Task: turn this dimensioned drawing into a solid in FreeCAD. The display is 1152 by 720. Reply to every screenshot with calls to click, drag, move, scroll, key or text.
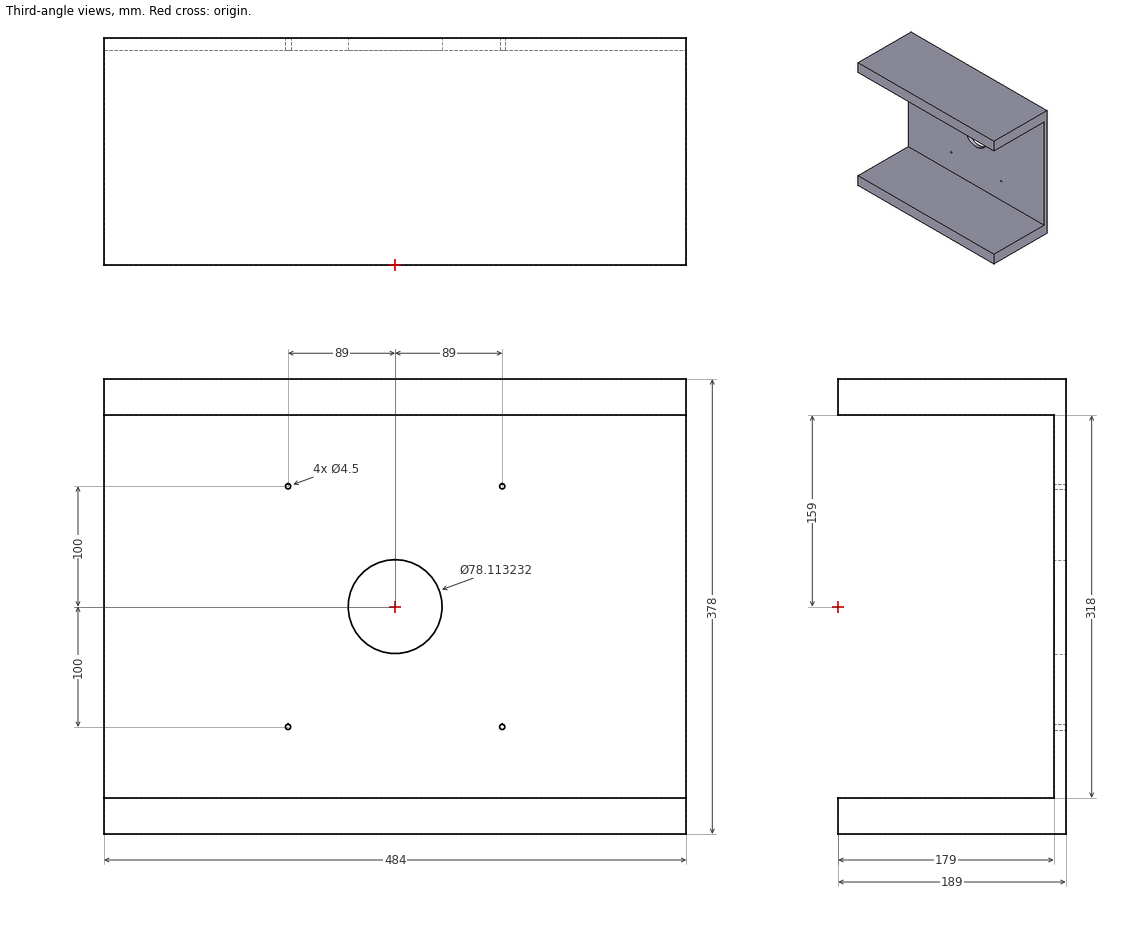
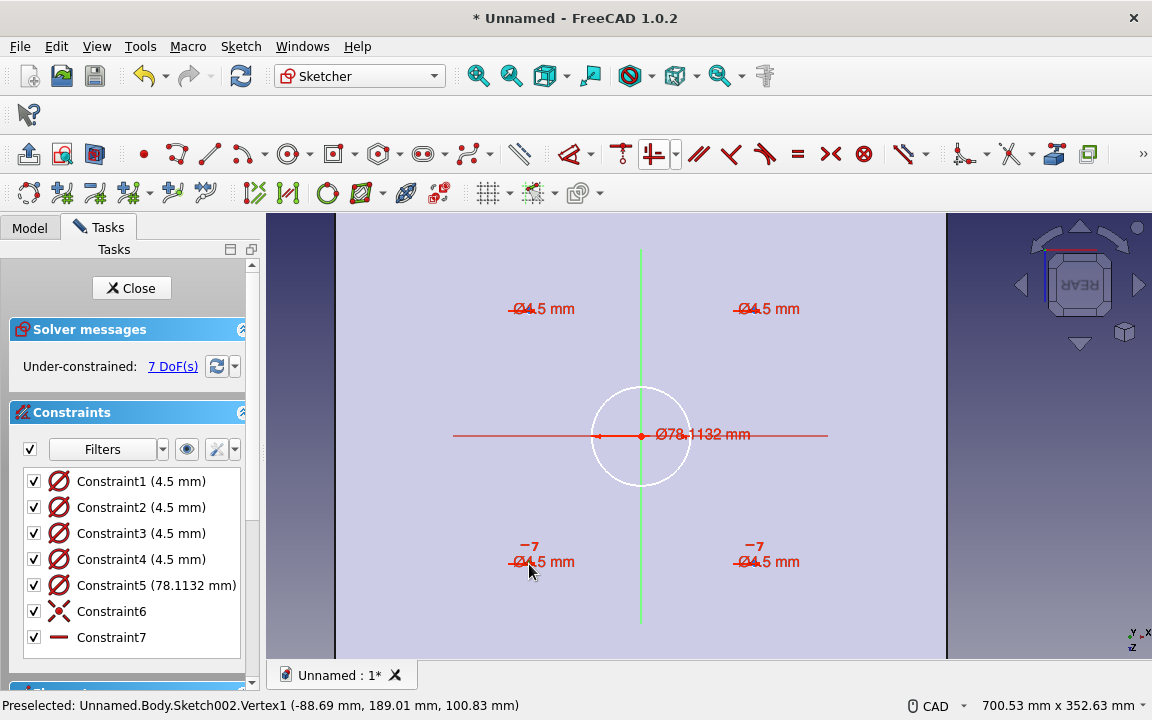
click(529, 311)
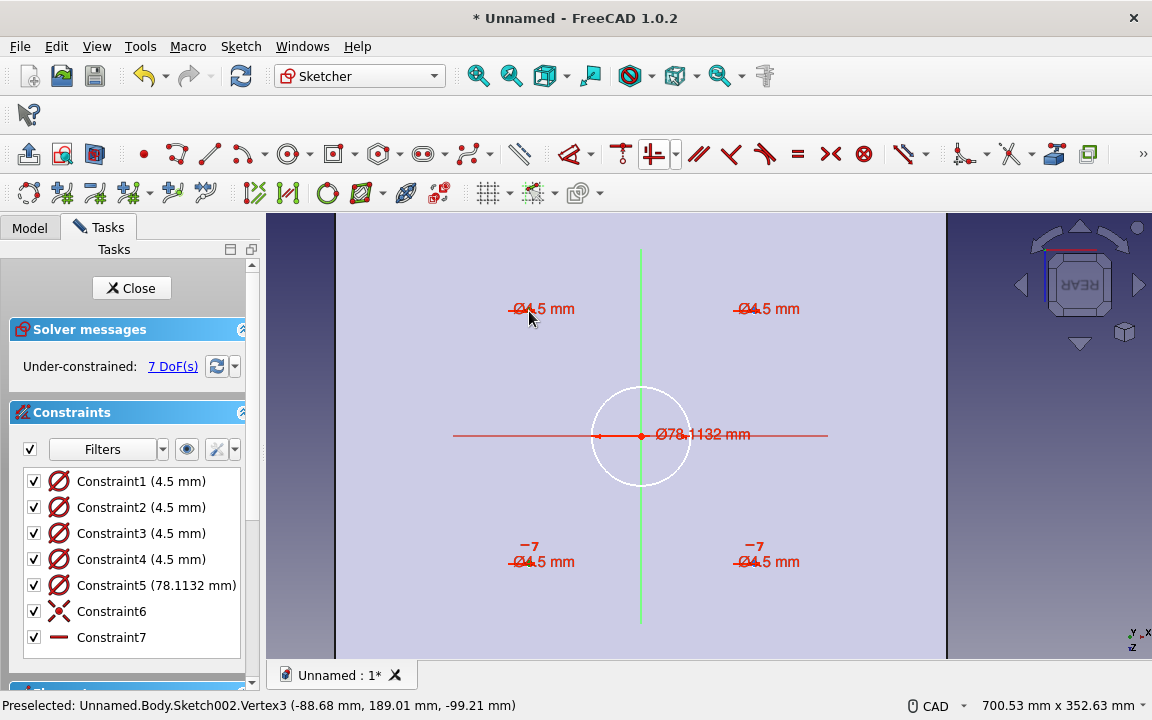
key(v)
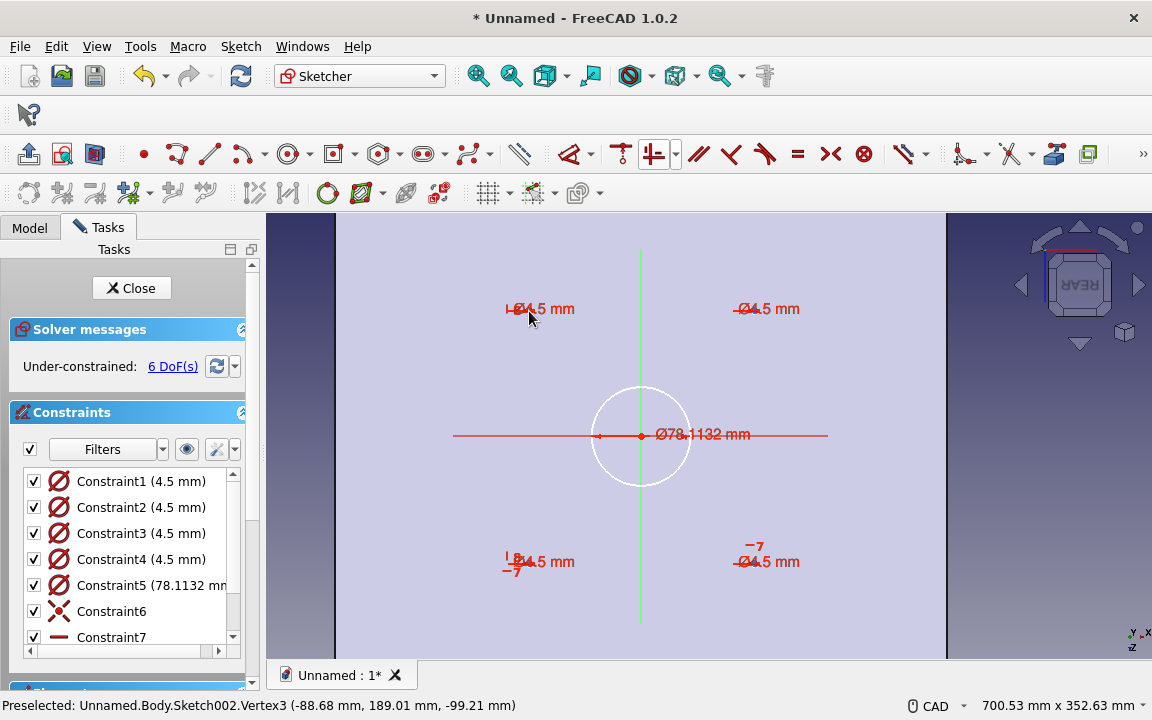
click(754, 564)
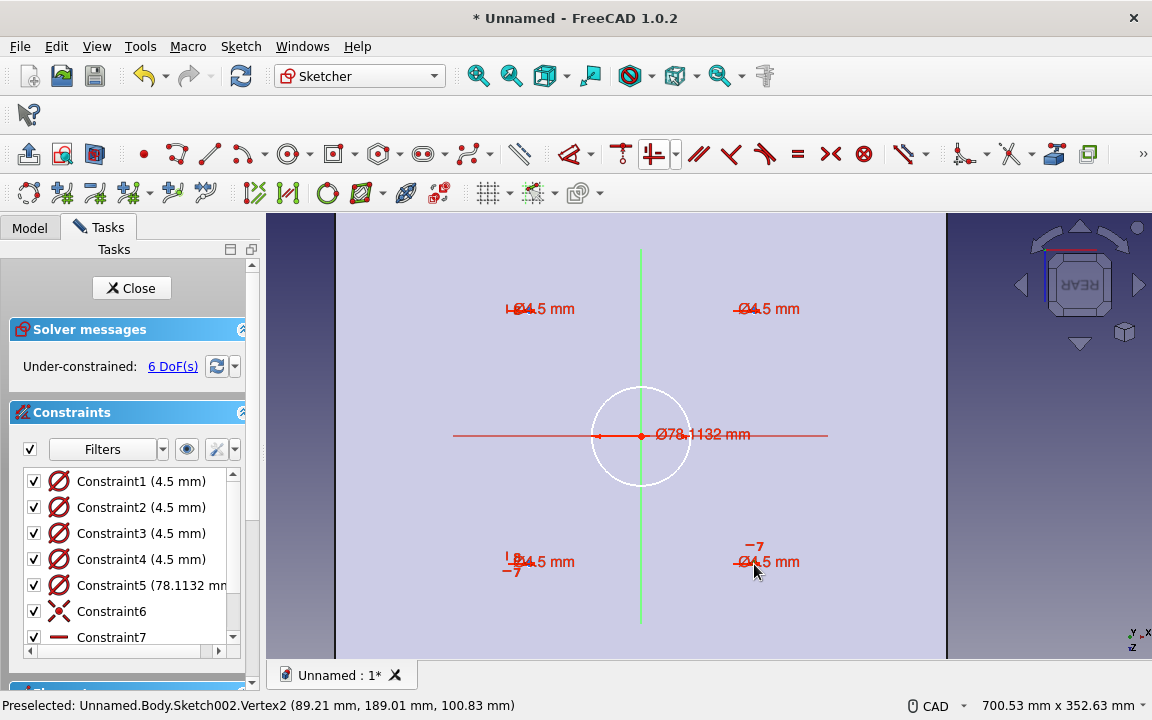
click(754, 311)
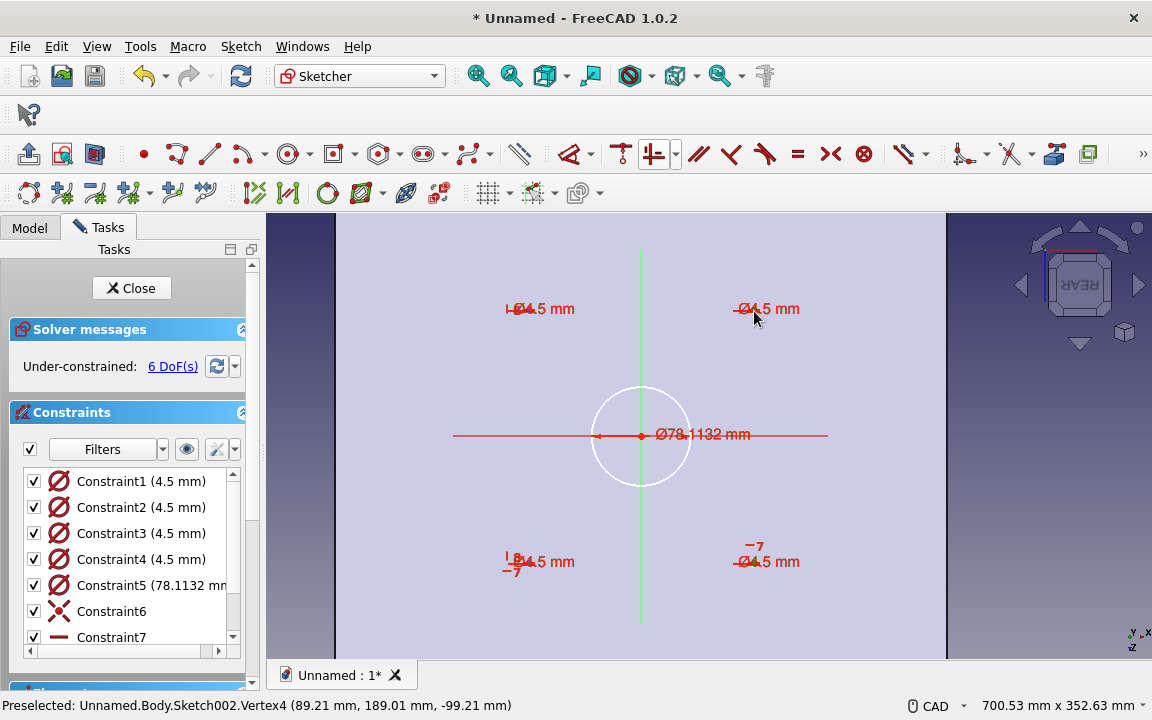
key(v)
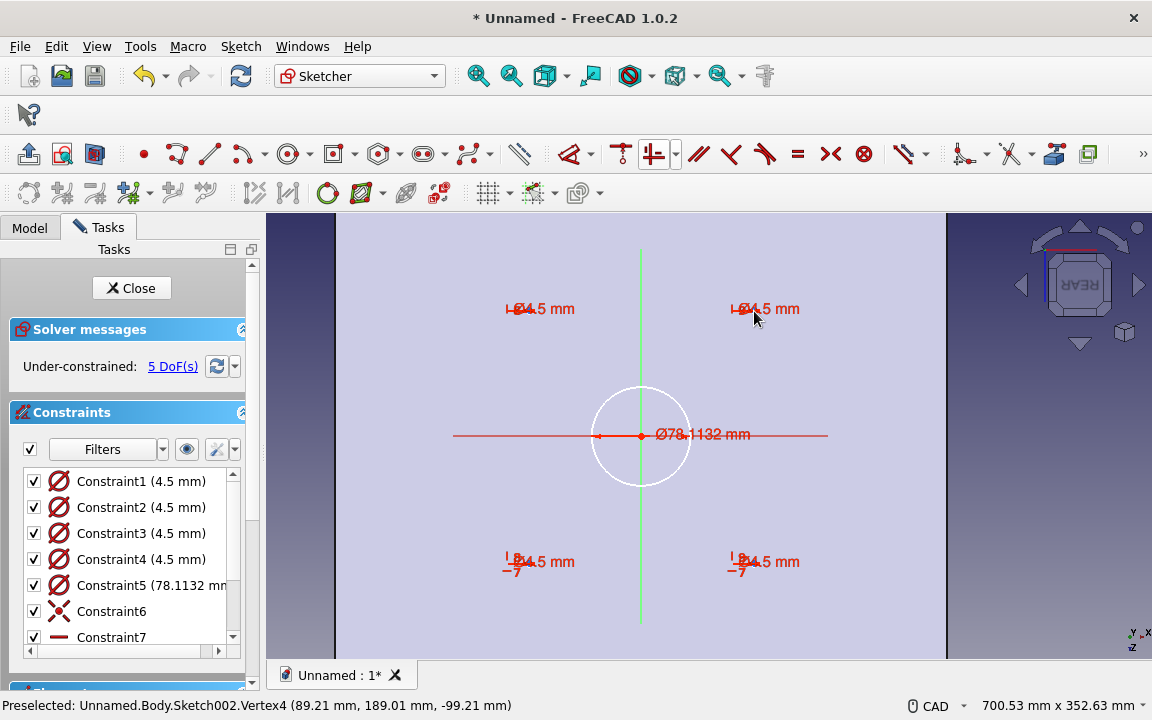
click(529, 311)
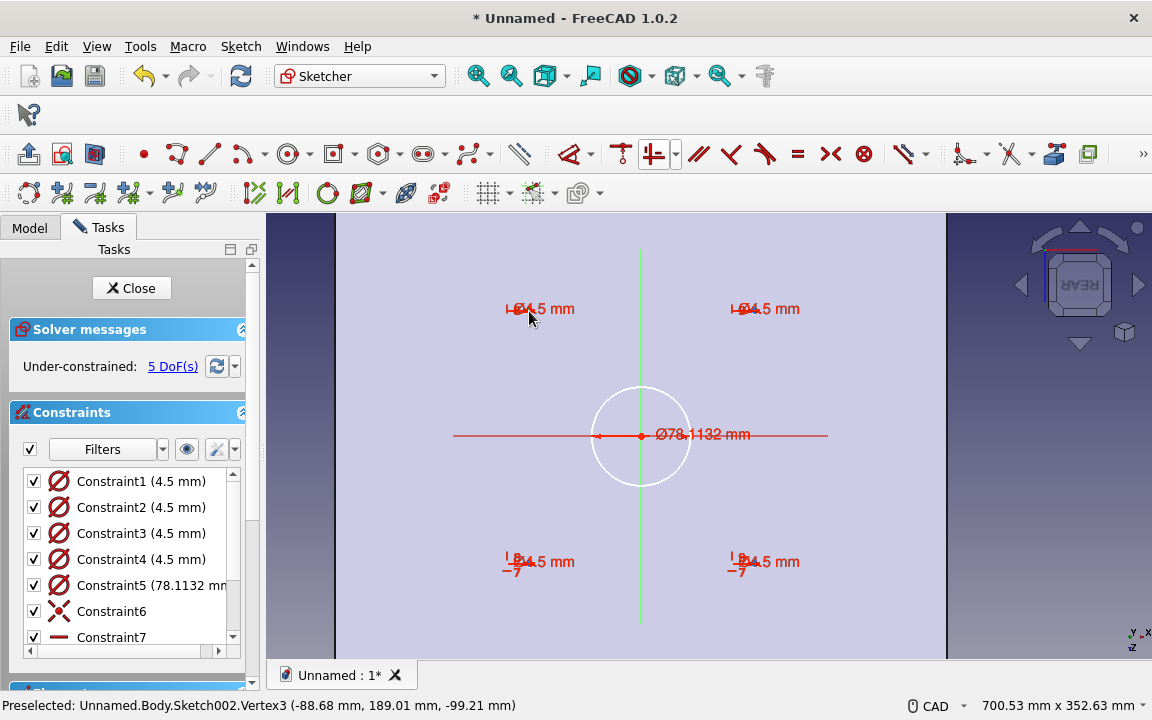
click(754, 311)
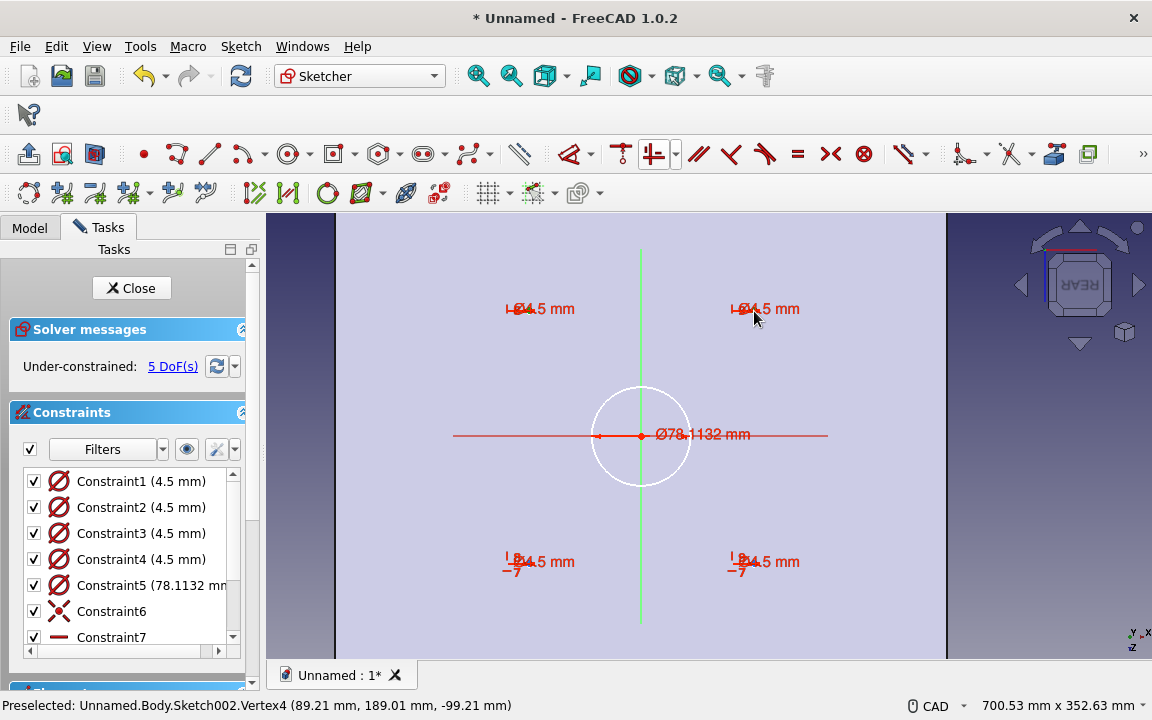
key(h)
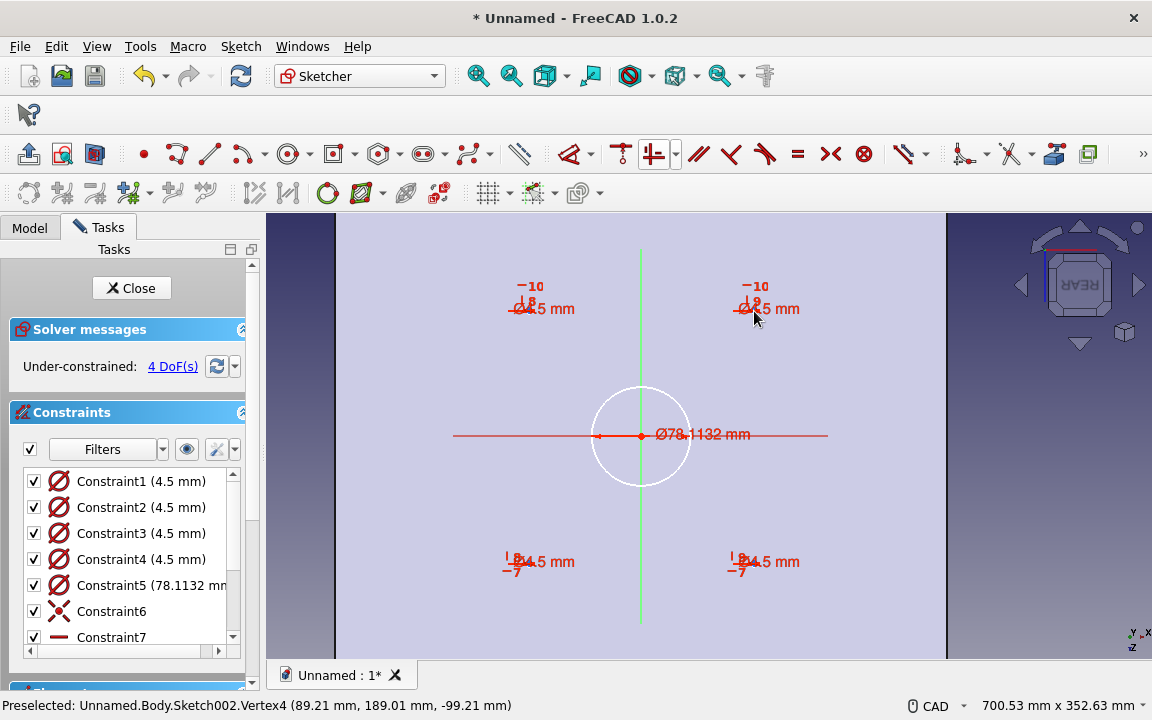
click(568, 154)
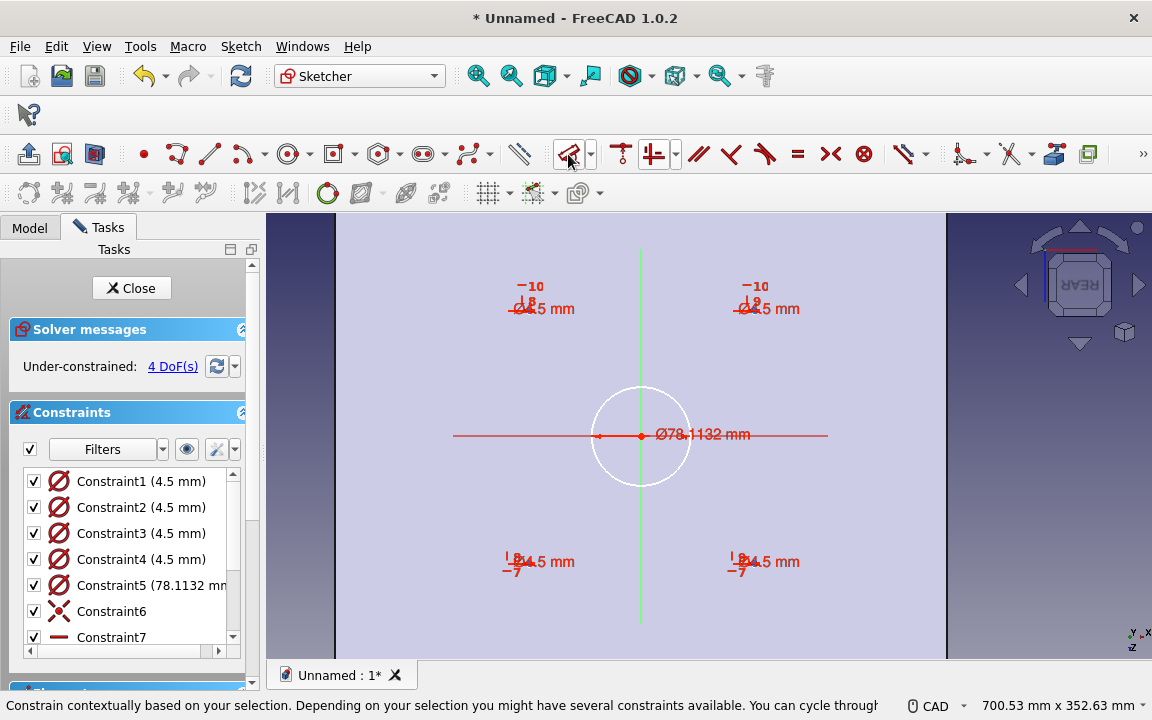
click(529, 564)
click(585, 598)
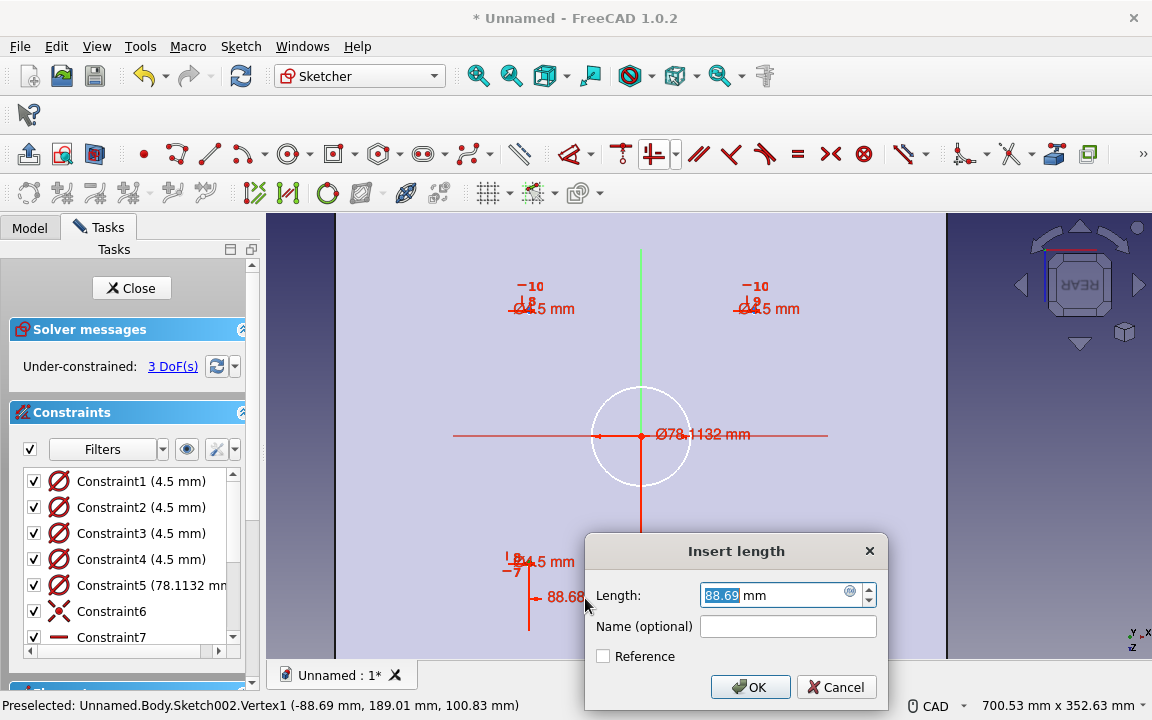
text(89)
key(Return)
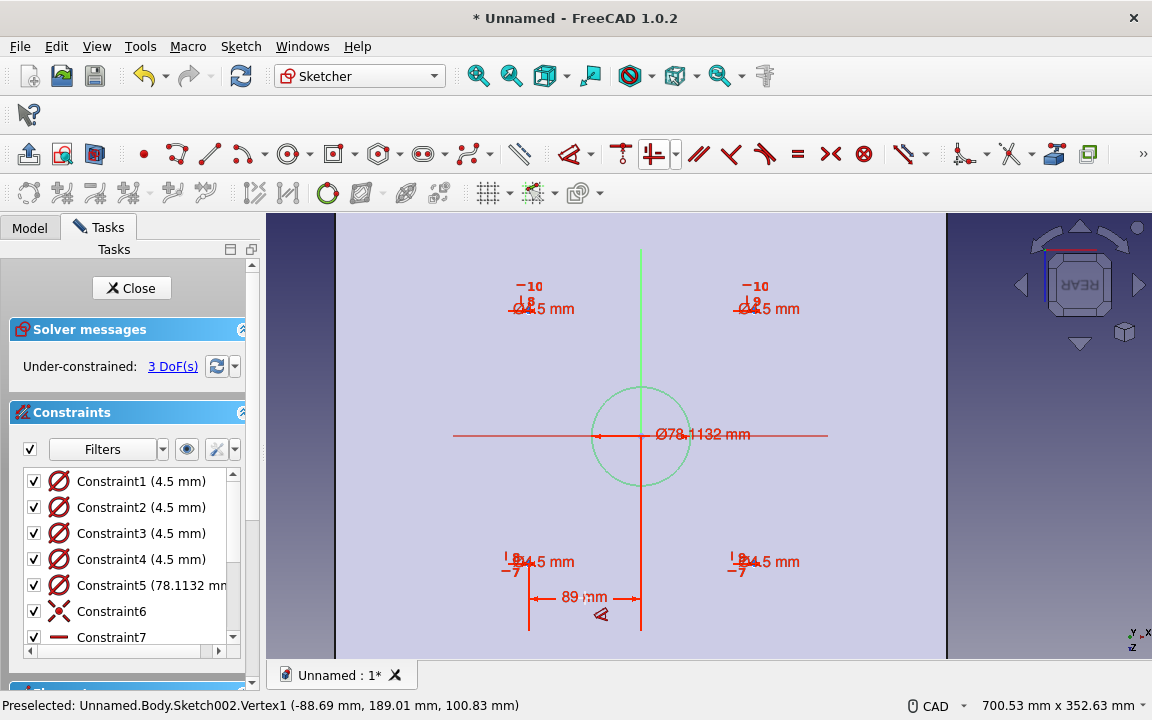
click(754, 564)
click(698, 598)